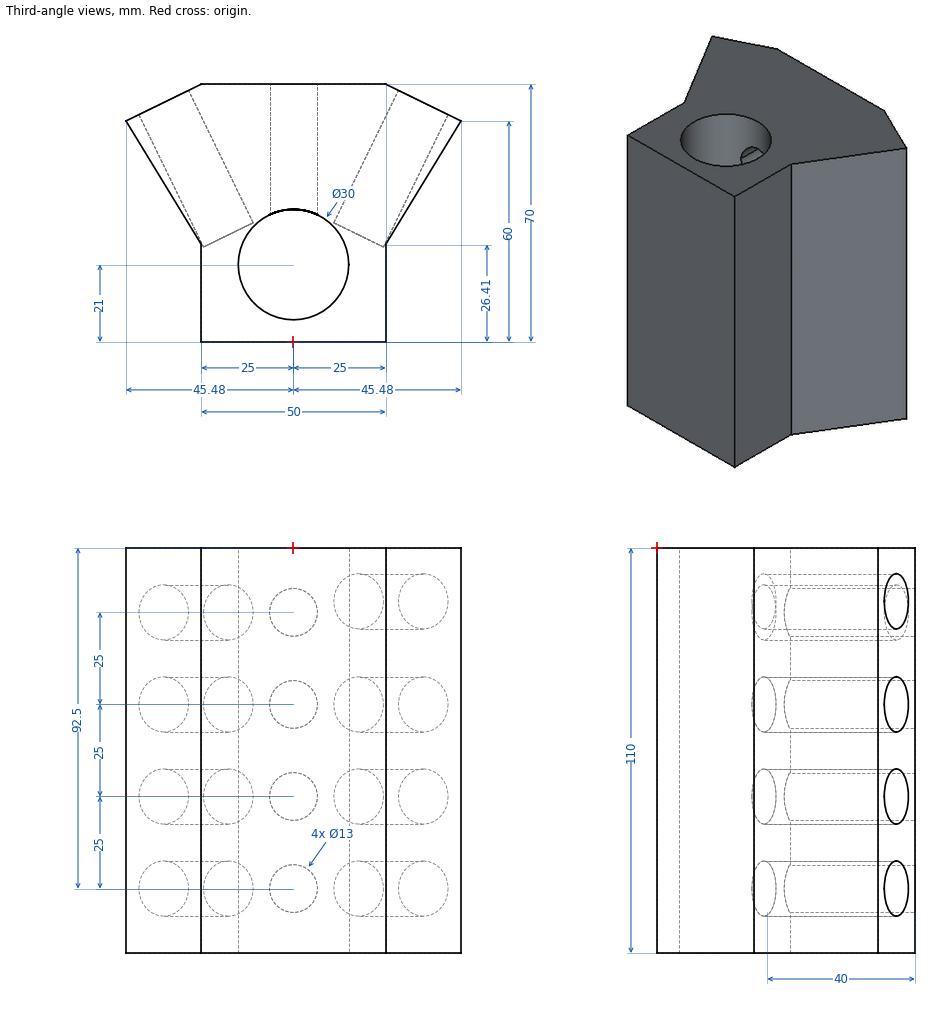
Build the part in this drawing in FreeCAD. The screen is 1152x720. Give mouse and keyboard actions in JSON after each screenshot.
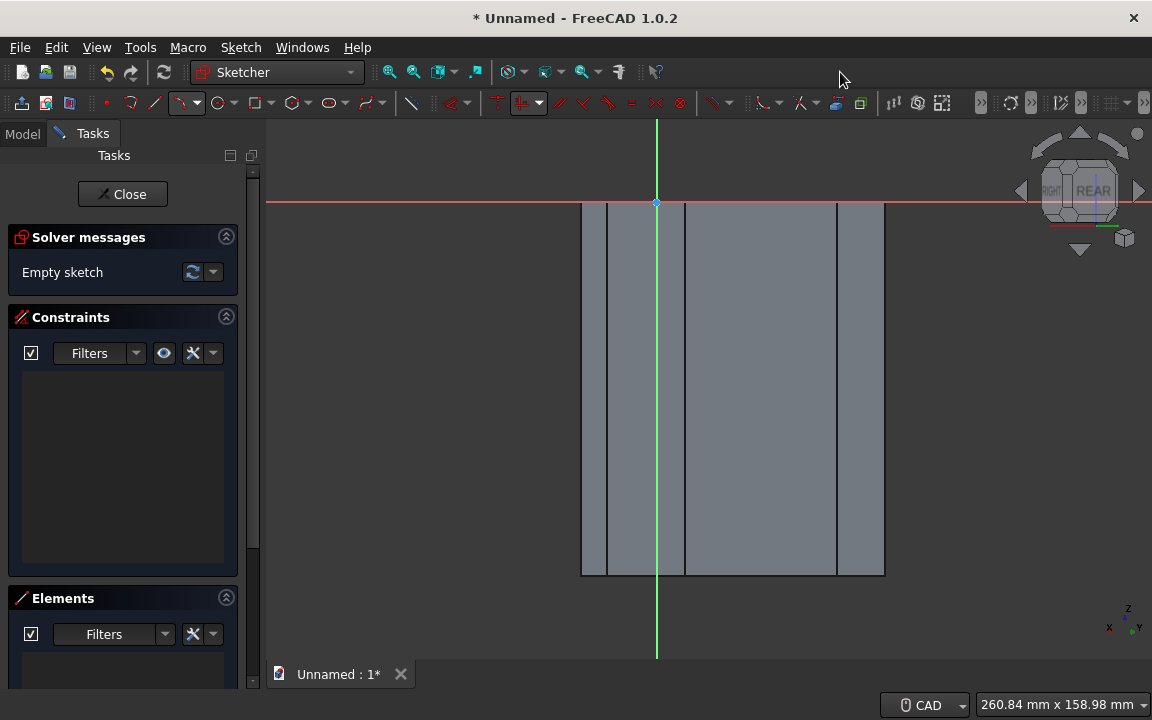
{"action": "key", "text": "g c"}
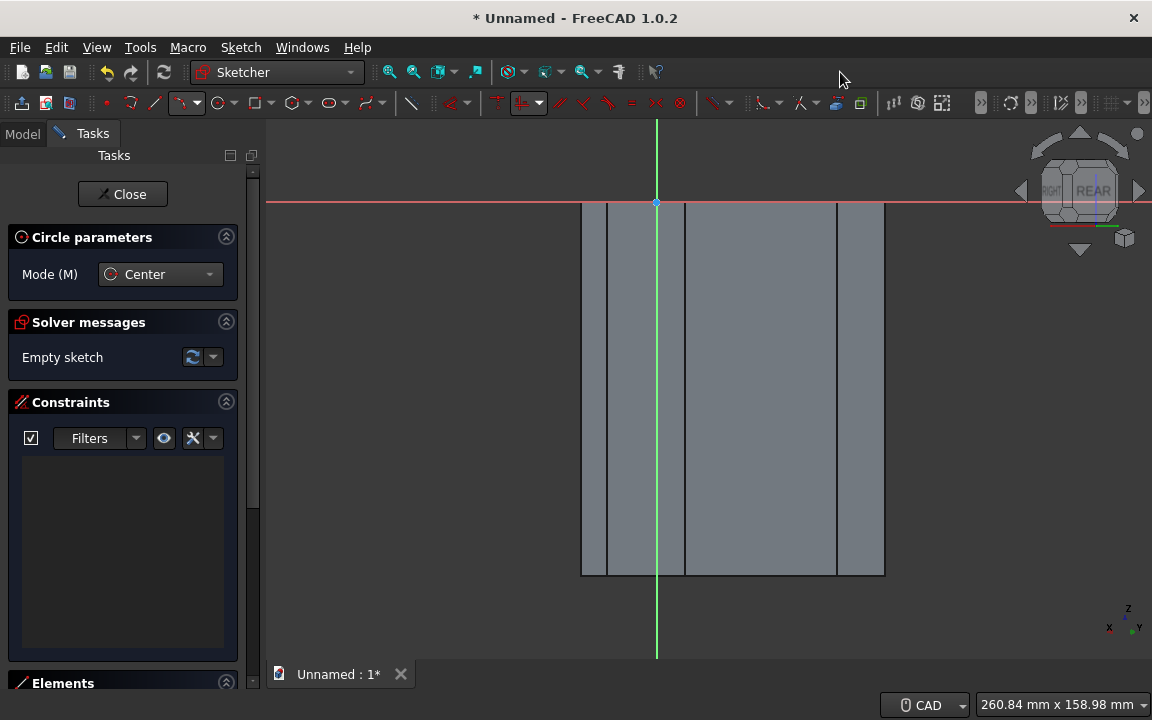
{"action": "scroll", "coordinate": [646, 516], "scroll_direction": "up", "scroll_amount": 2}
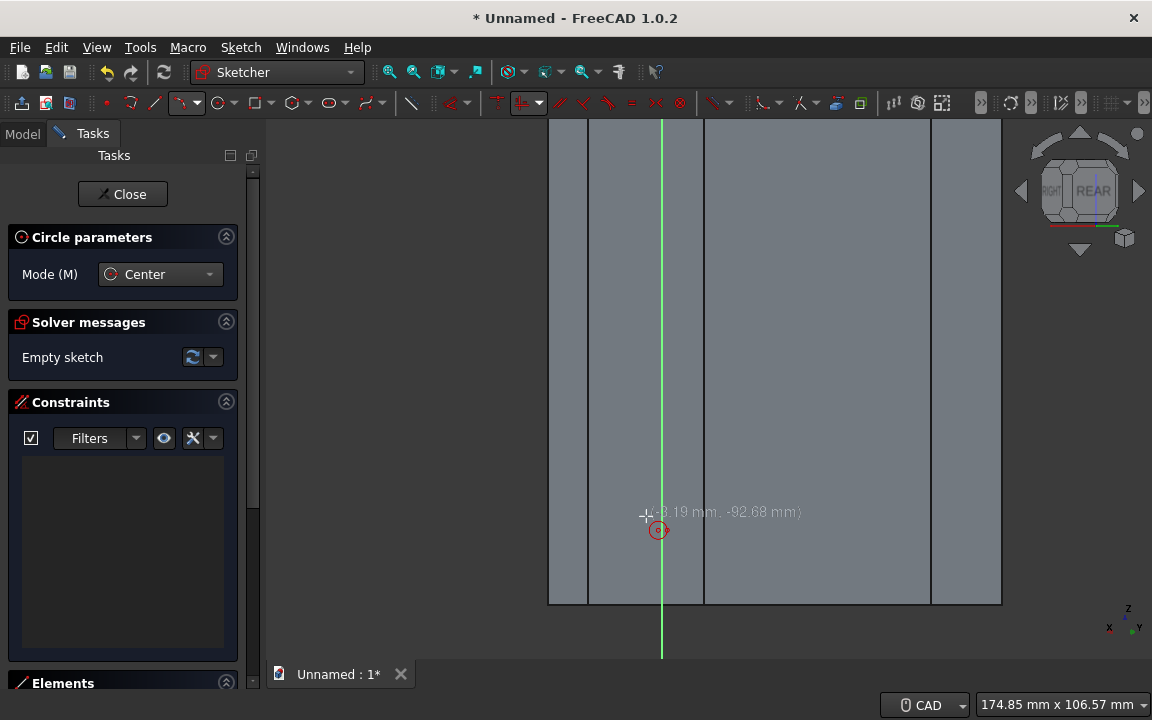
{"action": "left_click", "coordinate": [646, 516]}
{"action": "left_click", "coordinate": [619, 489]}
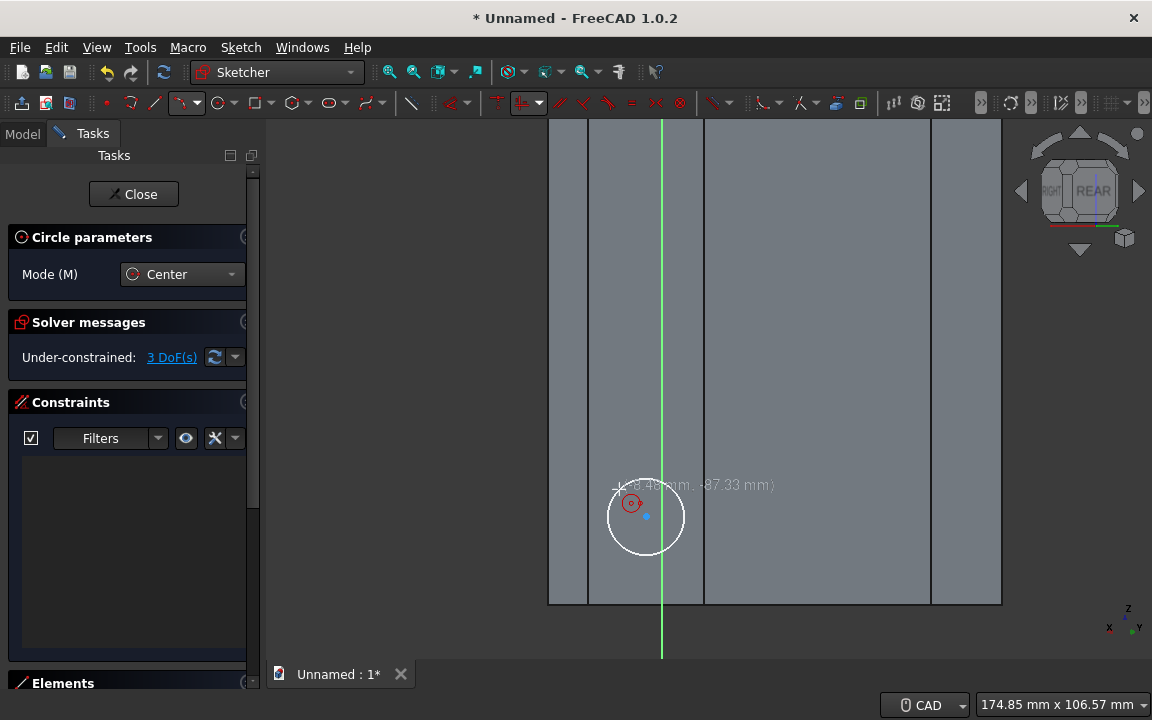
{"action": "left_click", "coordinate": [646, 390]}
{"action": "left_click", "coordinate": [619, 363]}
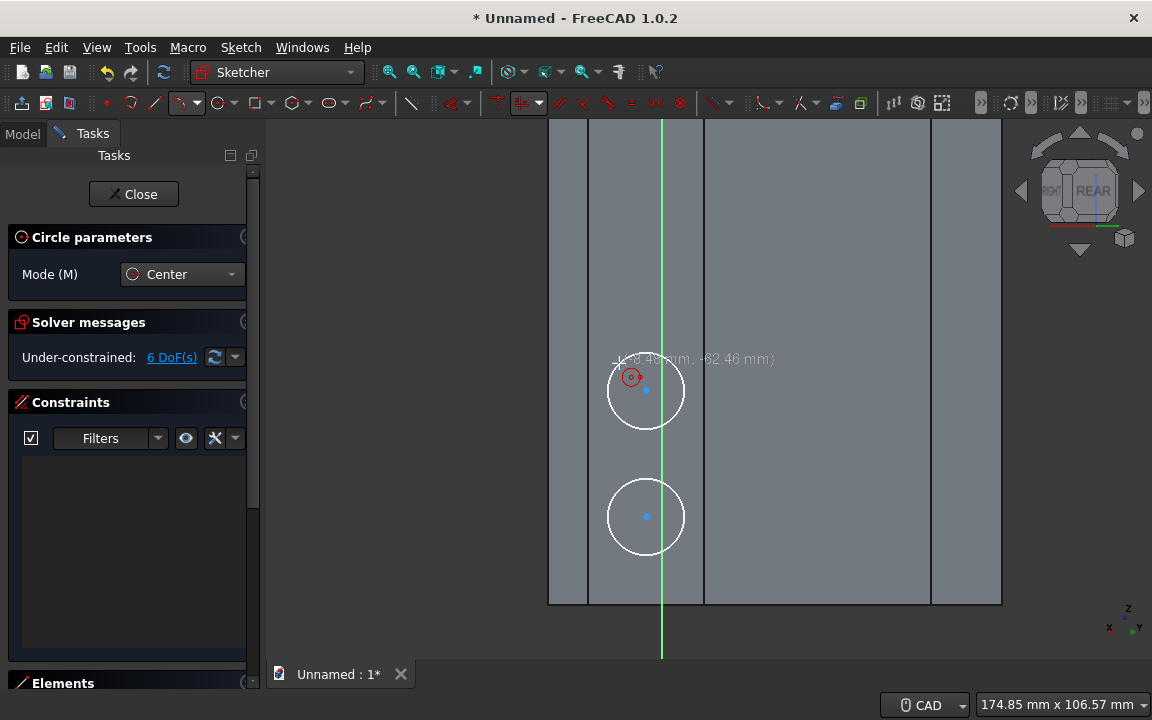
{"action": "left_click", "coordinate": [646, 263]}
{"action": "left_click", "coordinate": [619, 236]}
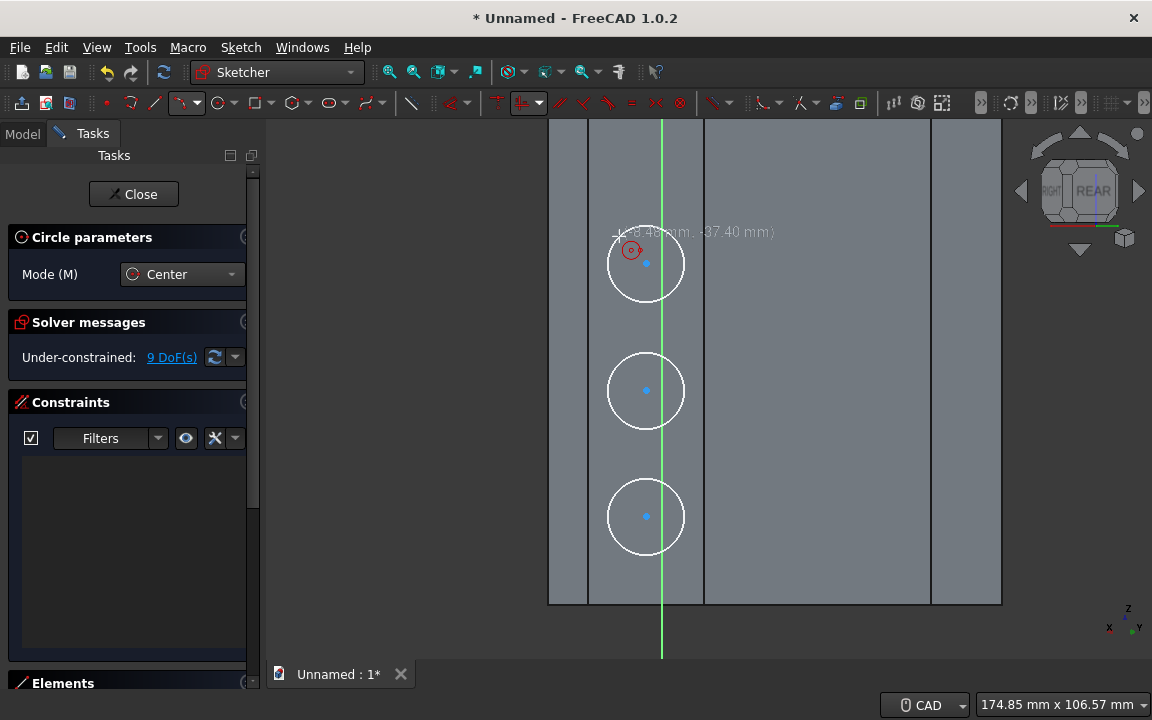
{"action": "scroll", "coordinate": [629, 568], "scroll_direction": "down", "scroll_amount": 2}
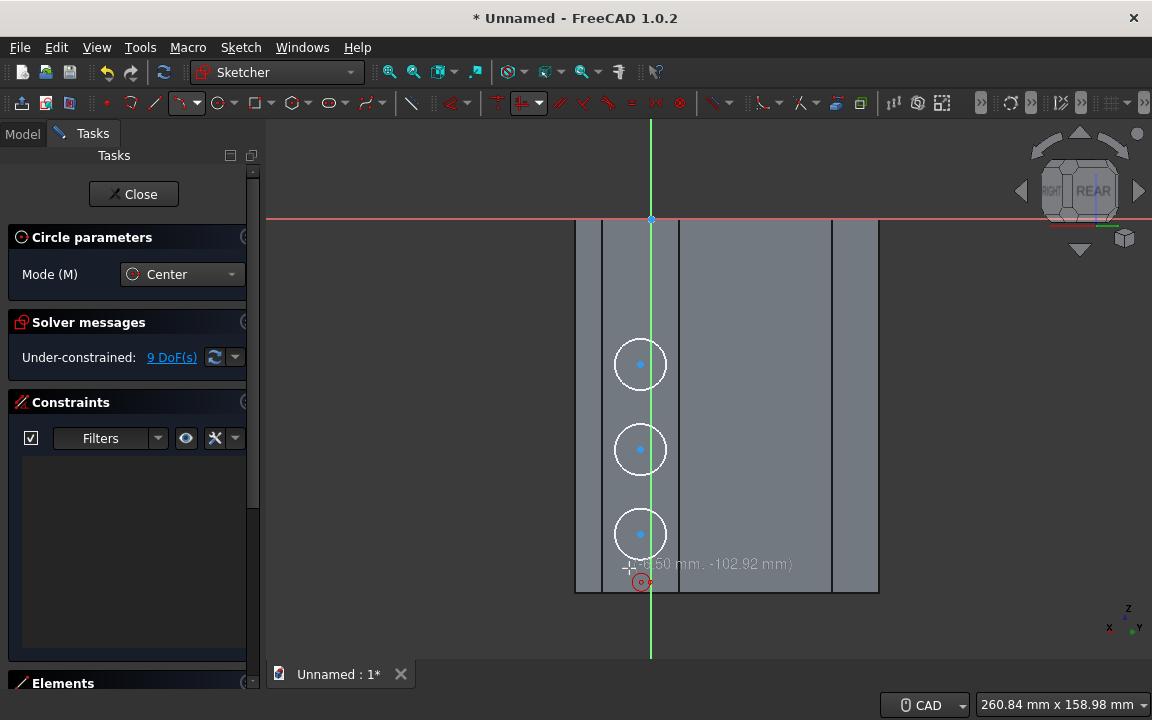
{"action": "scroll", "coordinate": [641, 269], "scroll_direction": "up", "scroll_amount": 2}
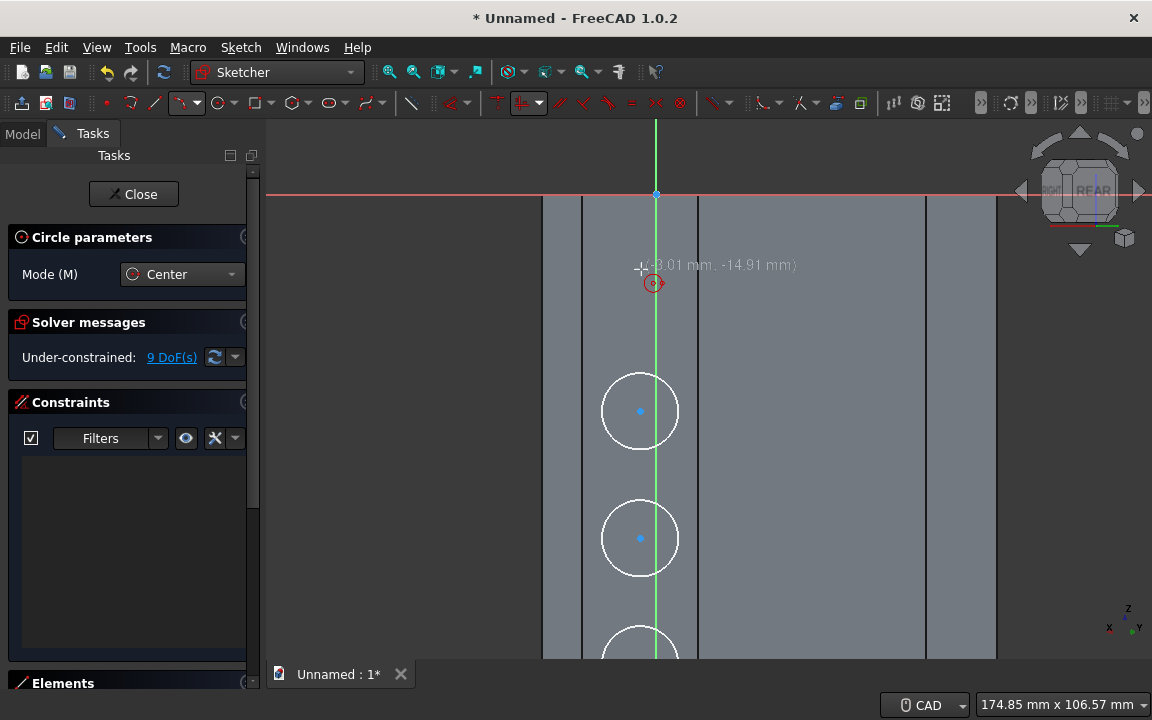
{"action": "left_click", "coordinate": [640, 268]}
{"action": "left_click", "coordinate": [613, 241]}
{"action": "key", "text": "Escape"}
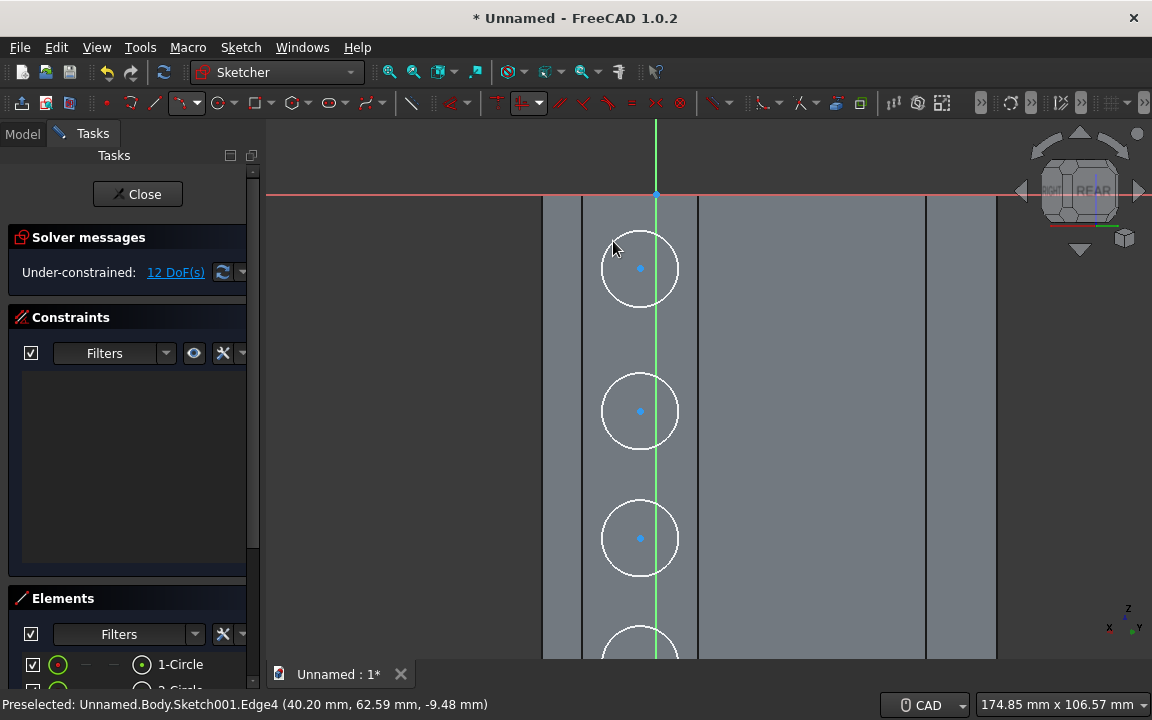
{"action": "left_click", "coordinate": [641, 626]}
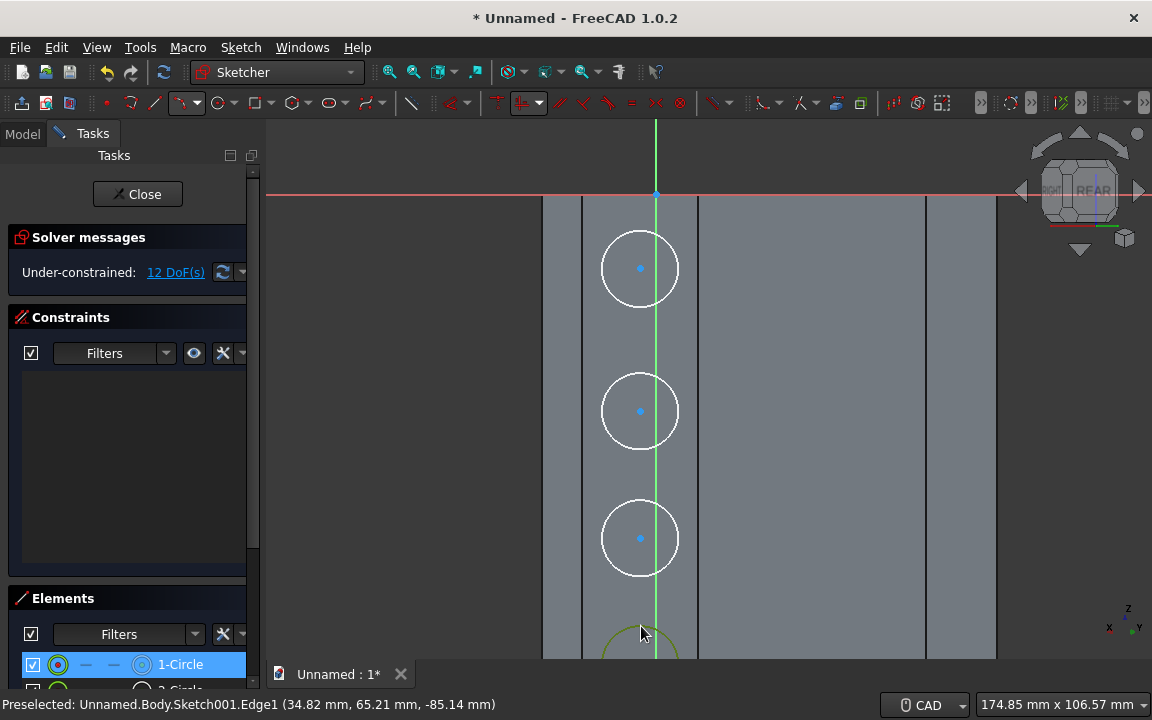
{"action": "scroll", "coordinate": [667, 511], "scroll_direction": "up", "scroll_amount": 2}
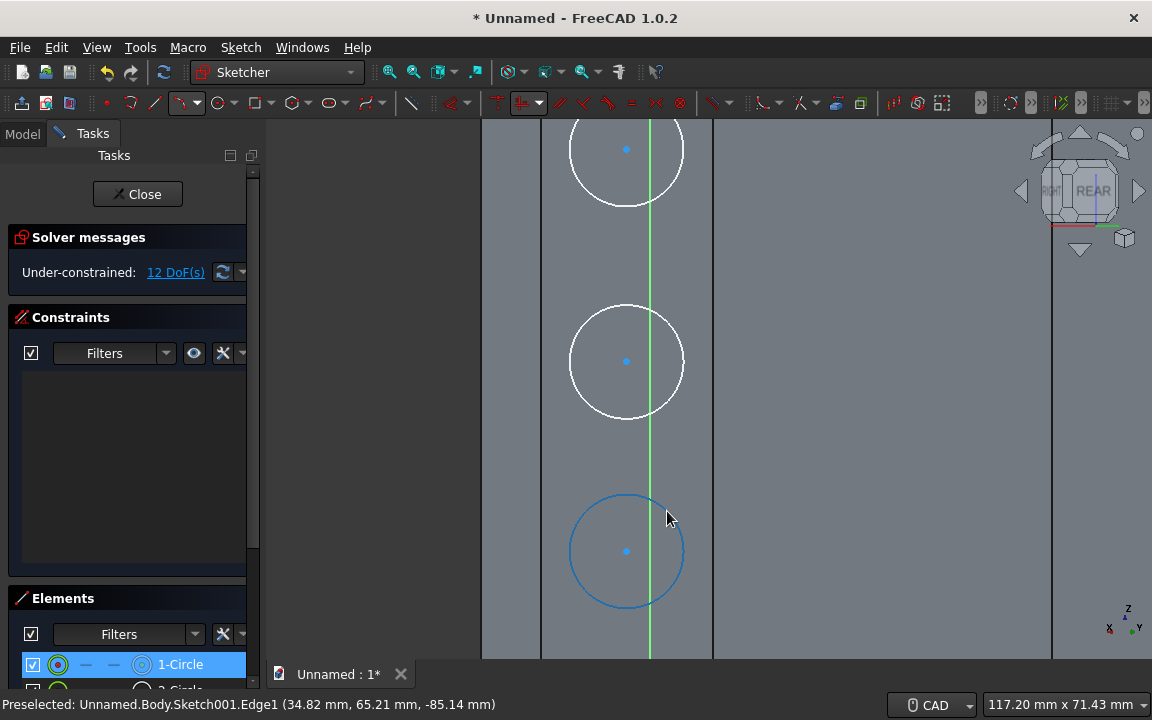
{"action": "left_click", "coordinate": [667, 511]}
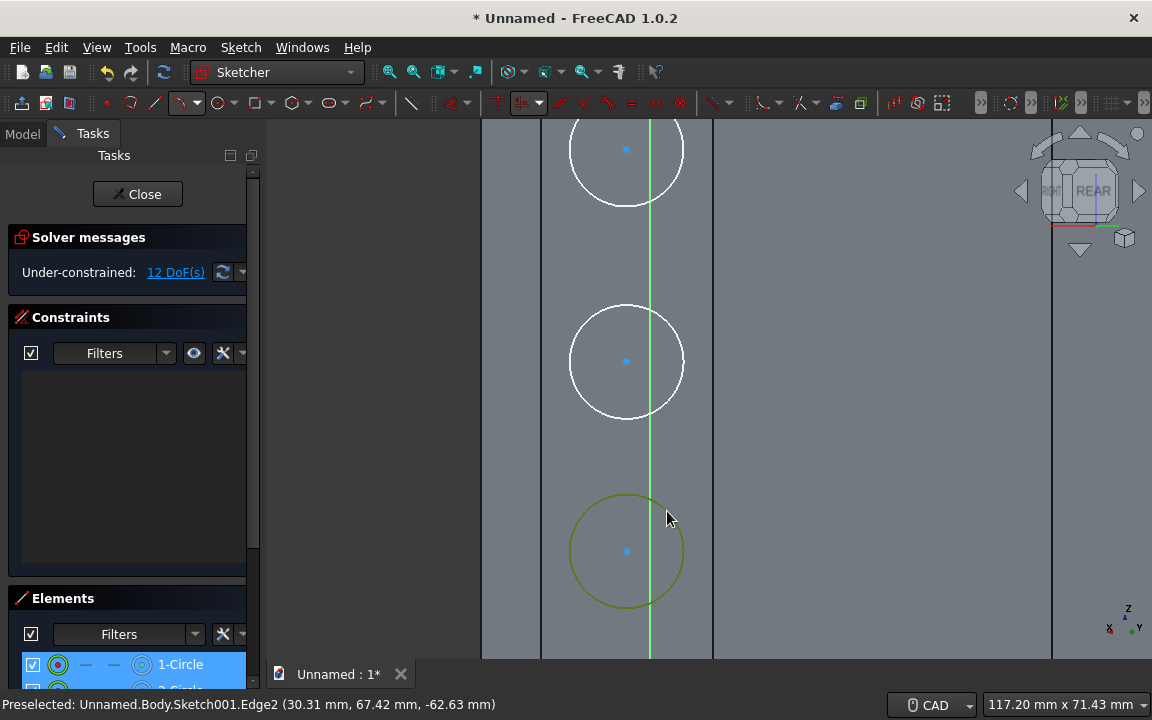
{"action": "left_click", "coordinate": [667, 322]}